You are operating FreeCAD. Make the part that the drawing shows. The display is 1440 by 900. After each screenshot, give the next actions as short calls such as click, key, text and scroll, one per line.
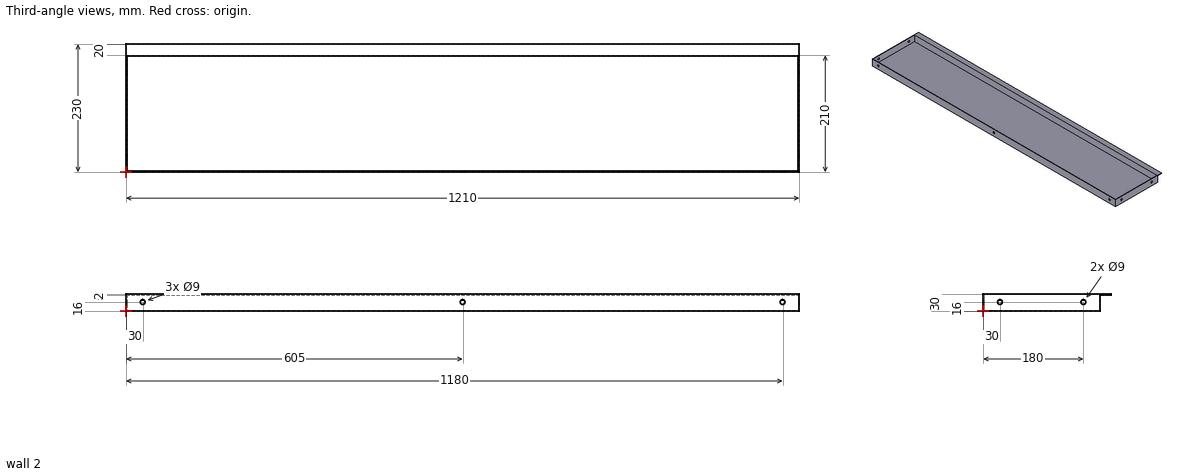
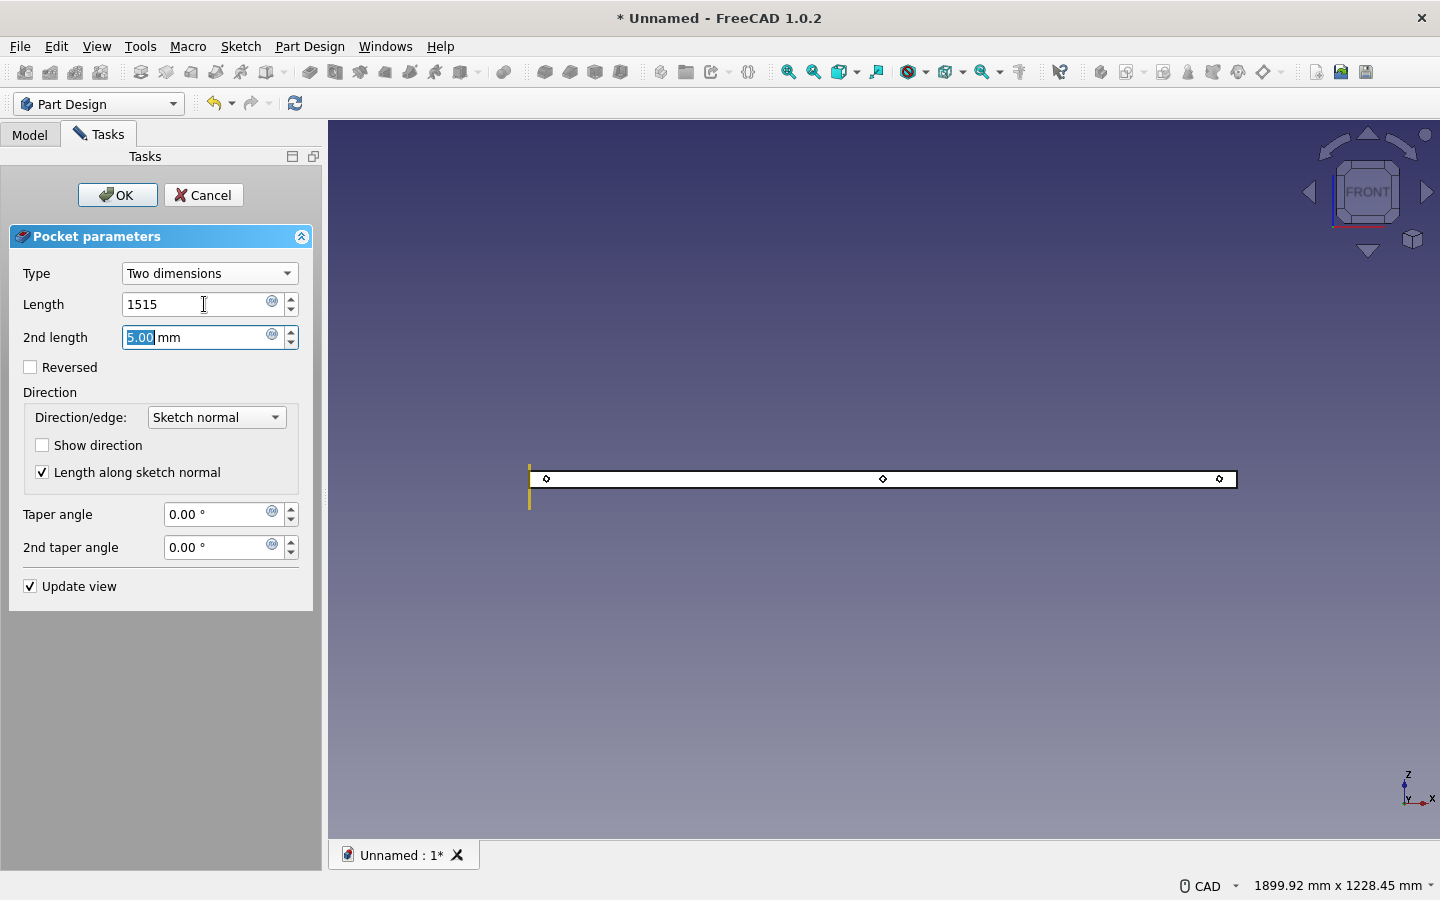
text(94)
key(Tab)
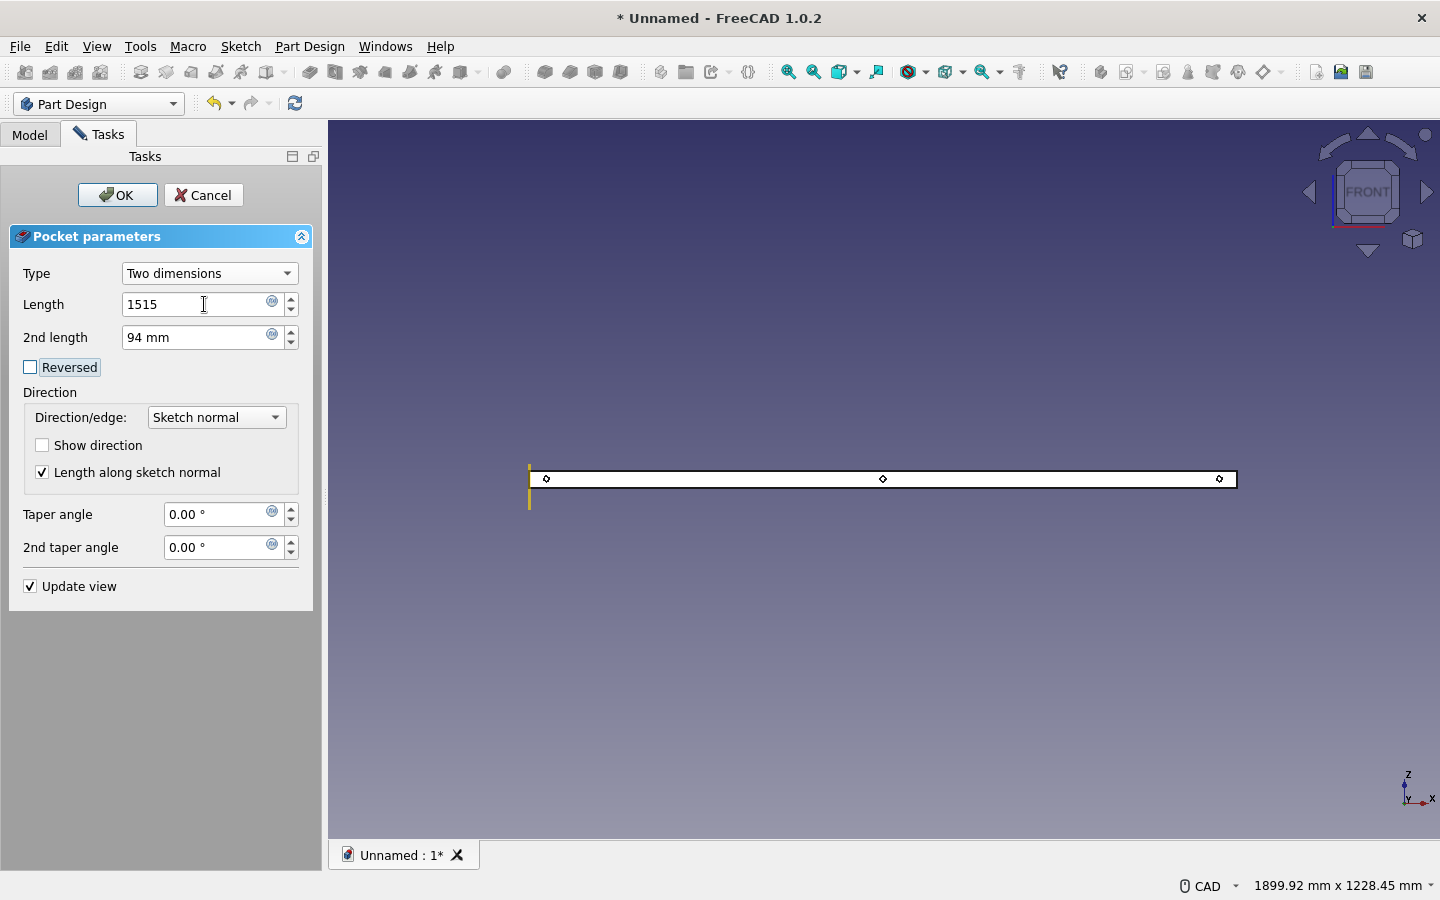
click(31, 367)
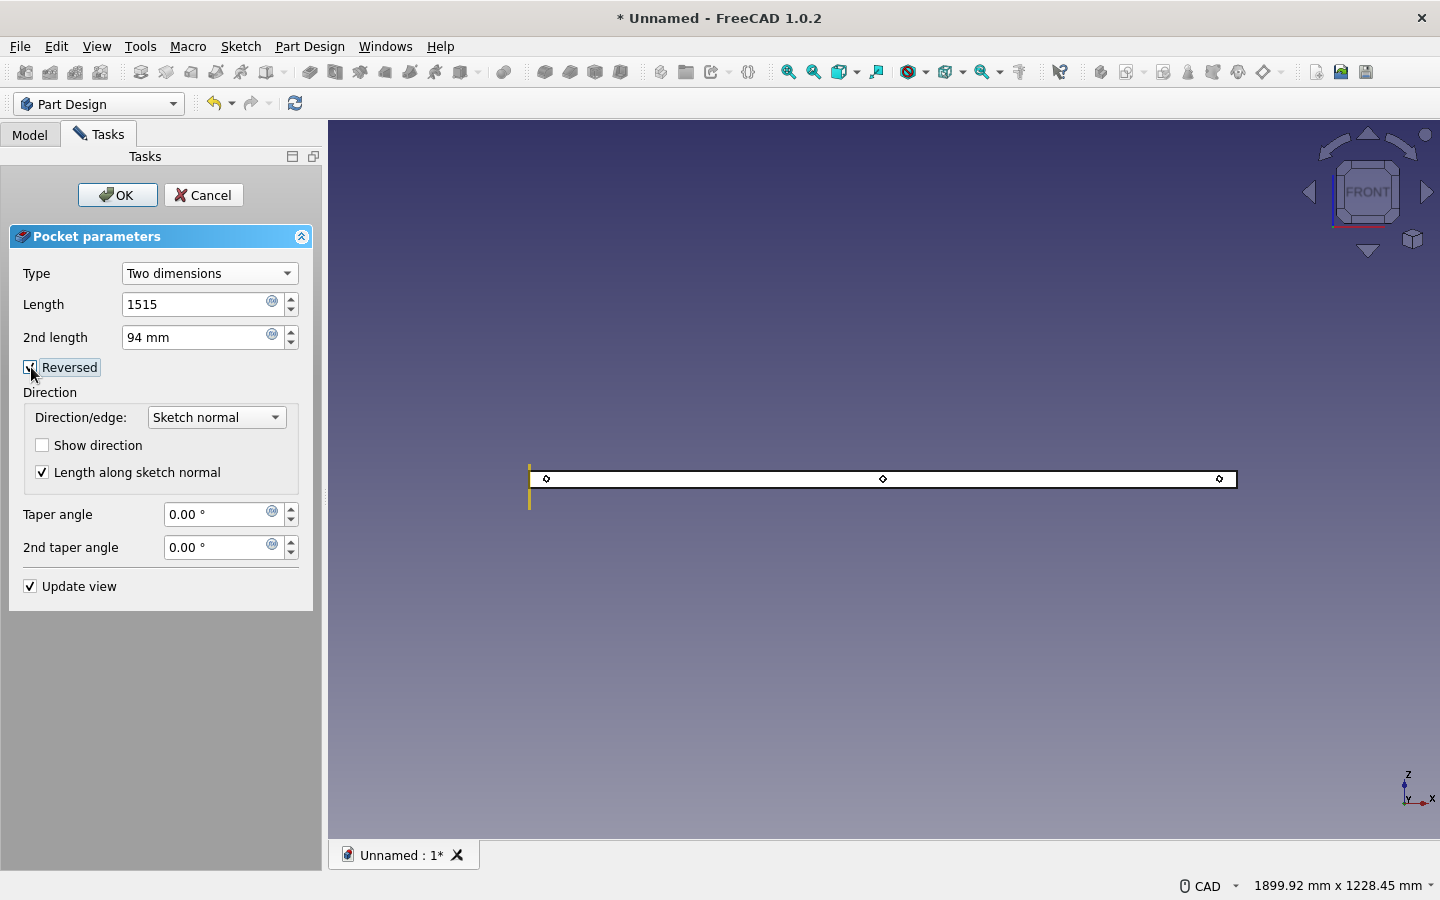
click(118, 195)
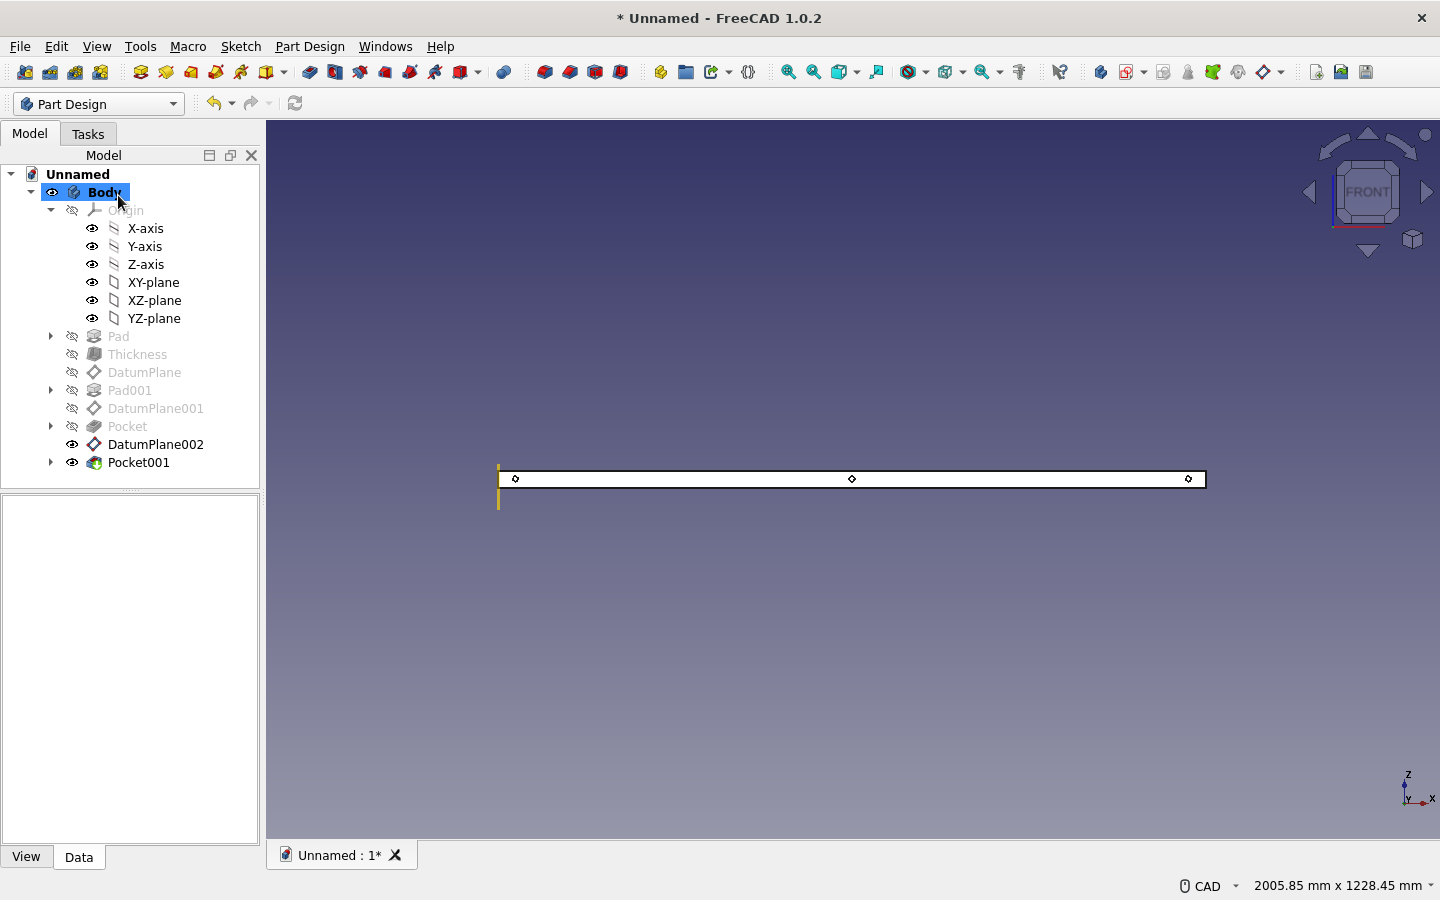
click(117, 444)
key(space)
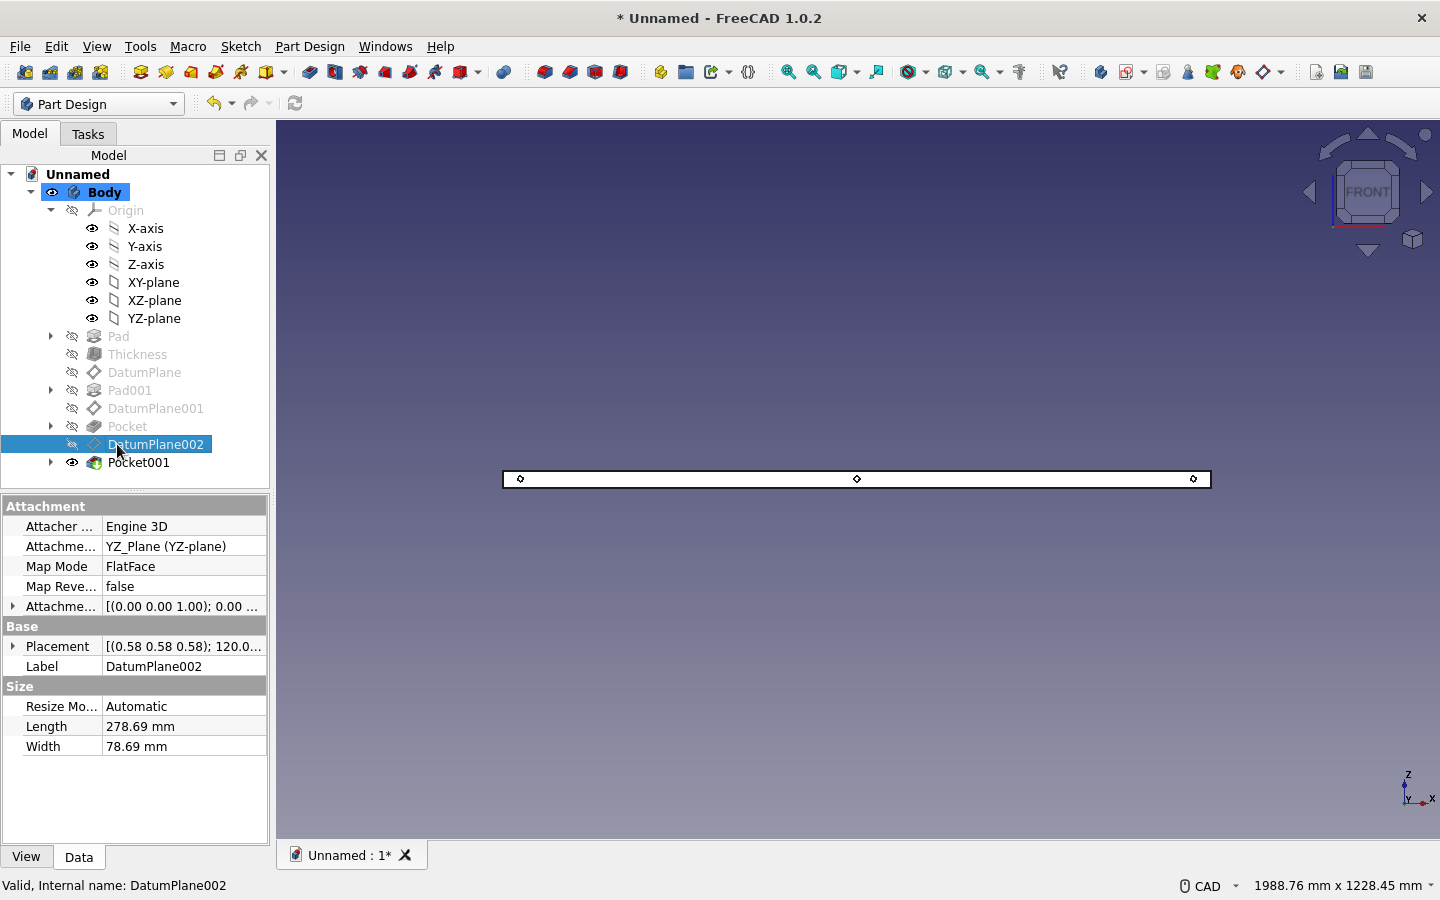
key(0)